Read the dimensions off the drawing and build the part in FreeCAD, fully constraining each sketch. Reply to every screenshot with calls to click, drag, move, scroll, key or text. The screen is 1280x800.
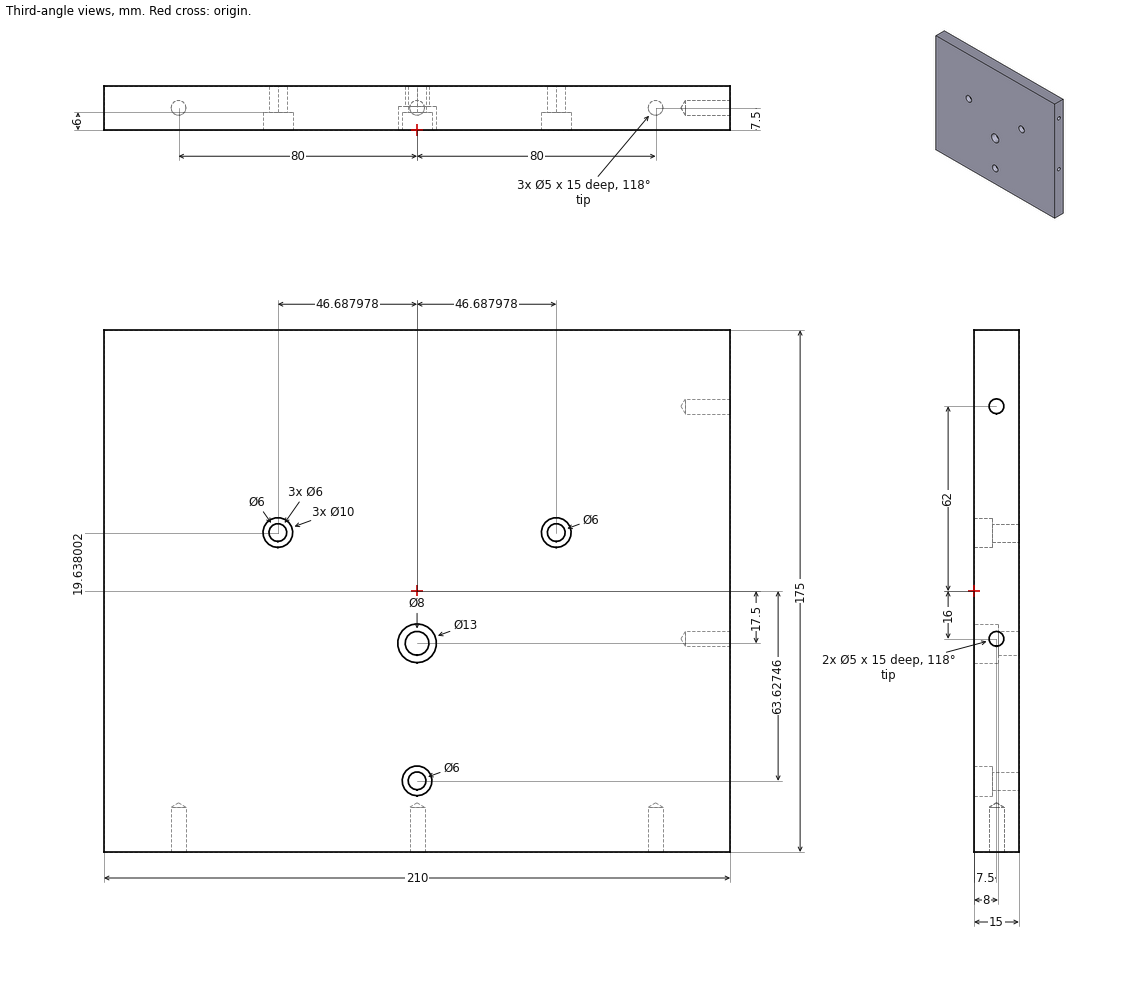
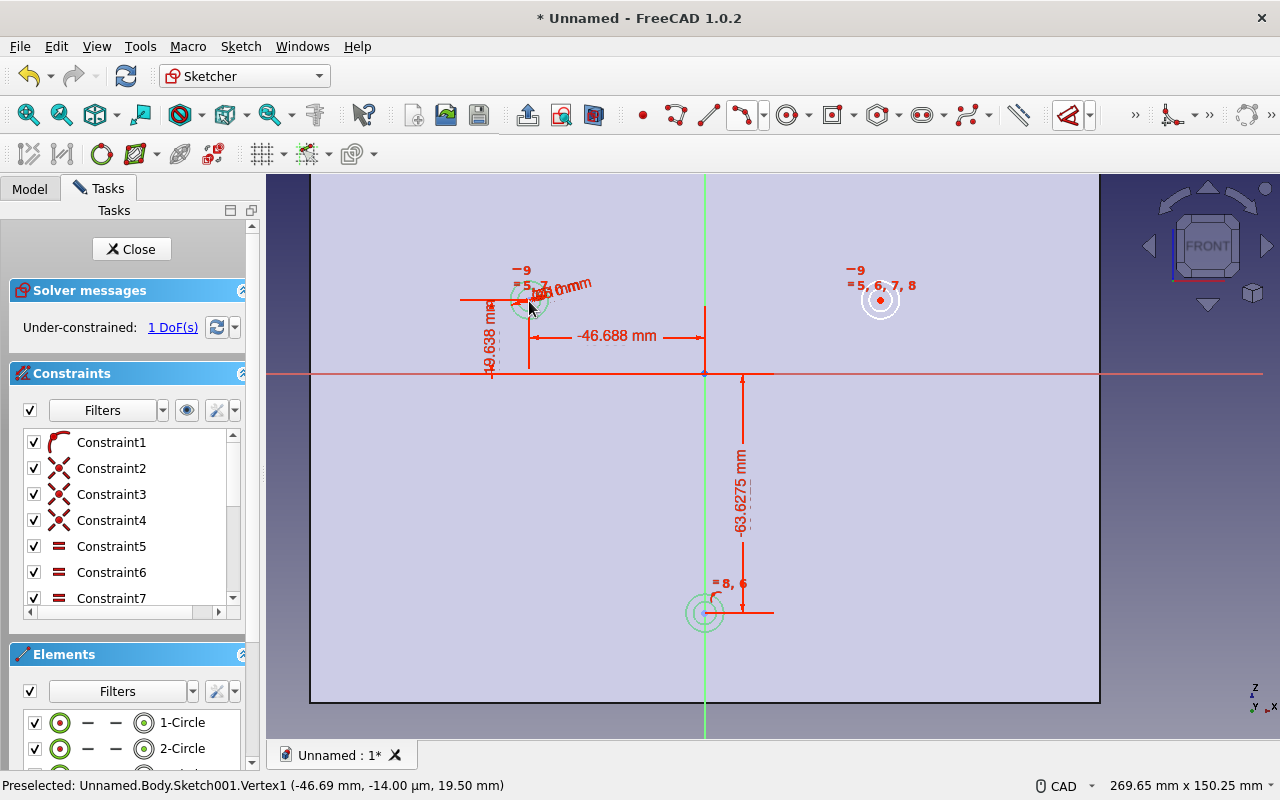
click(881, 300)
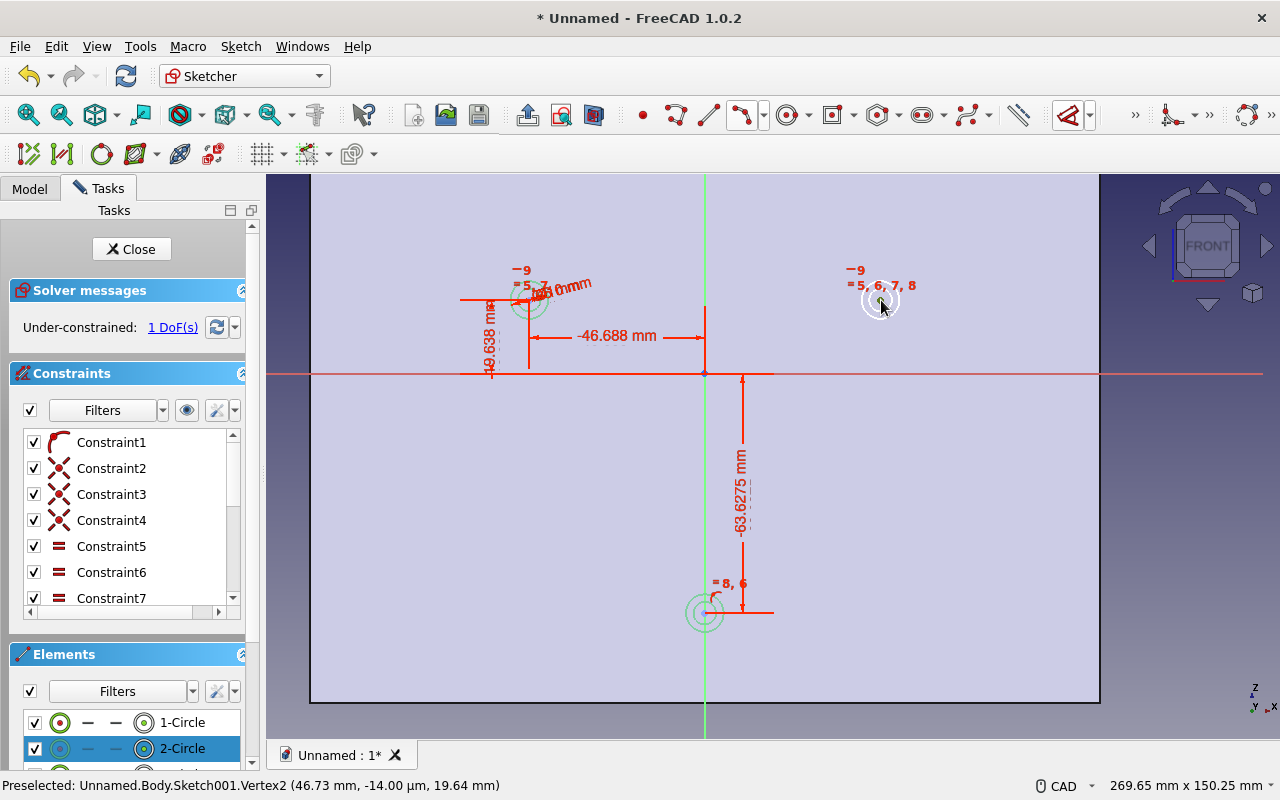
key(l)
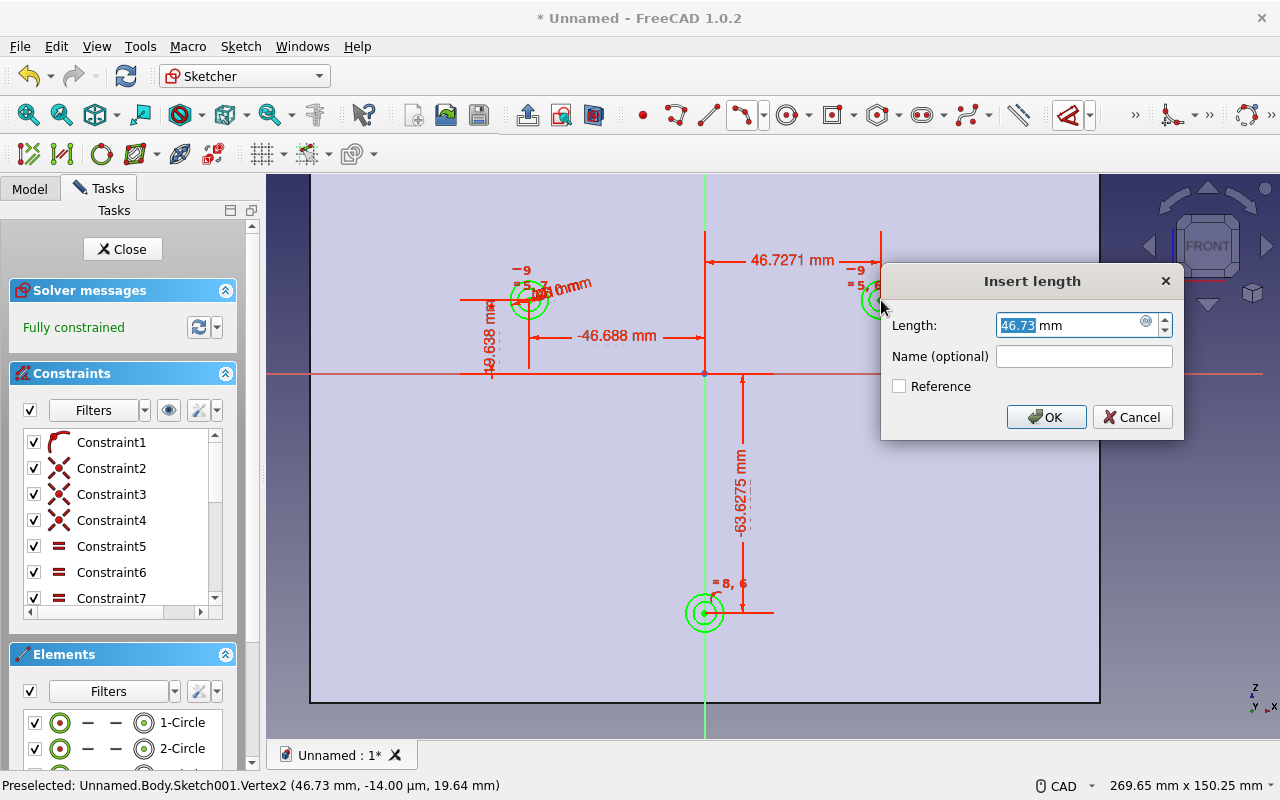
text(46.687978)
key(Return)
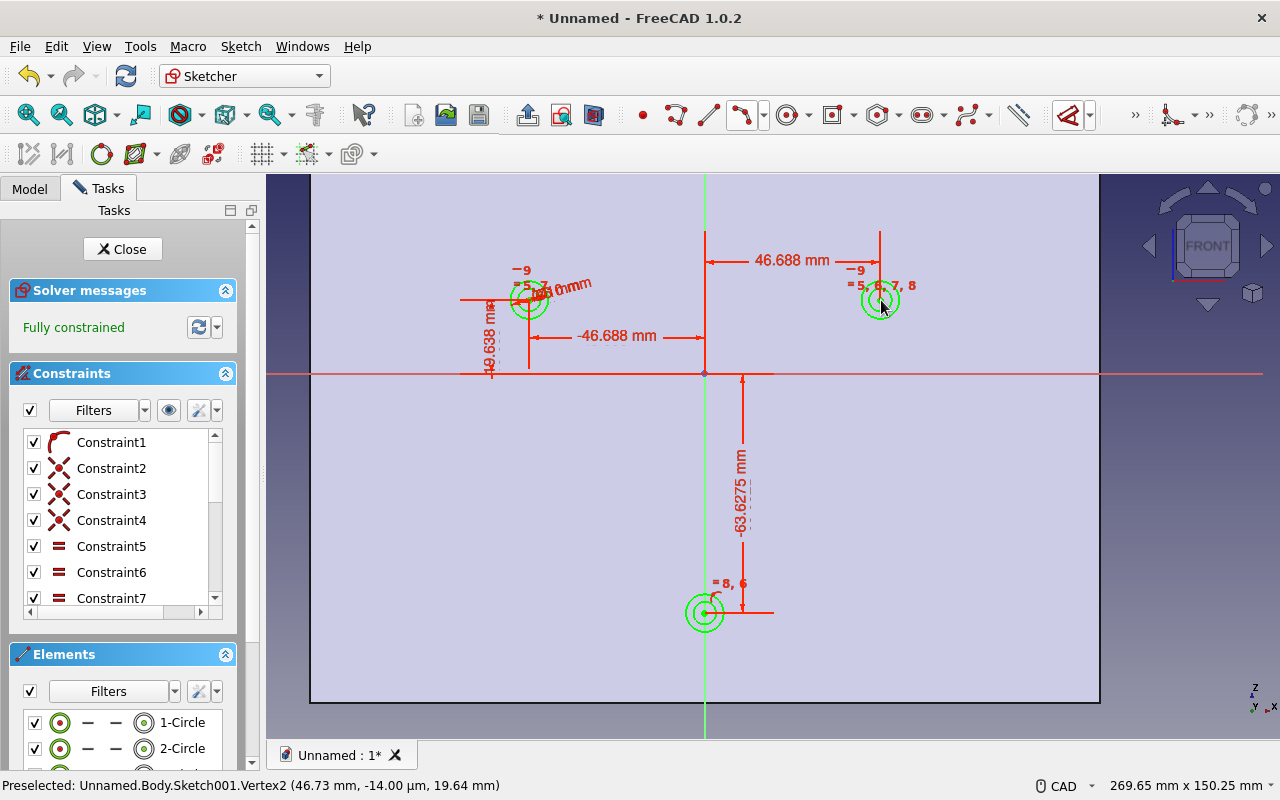
click(123, 249)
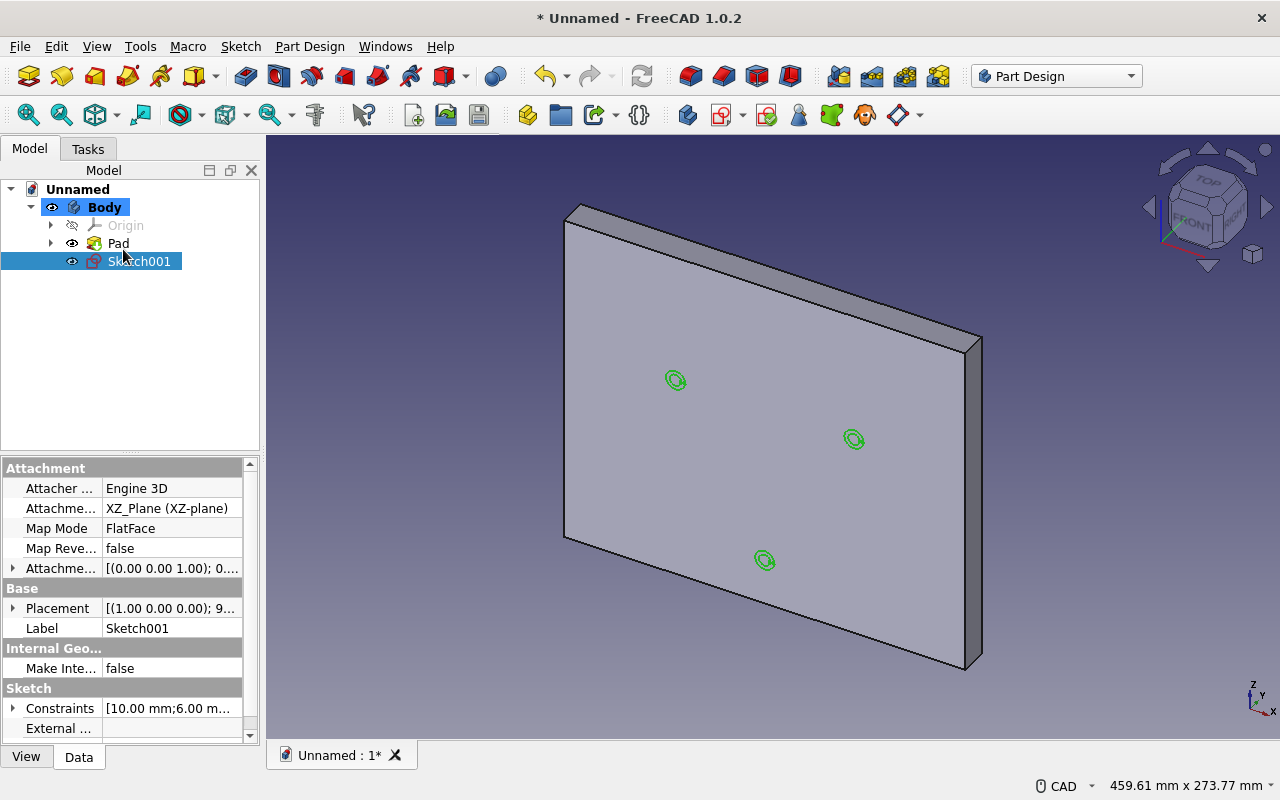
click(246, 76)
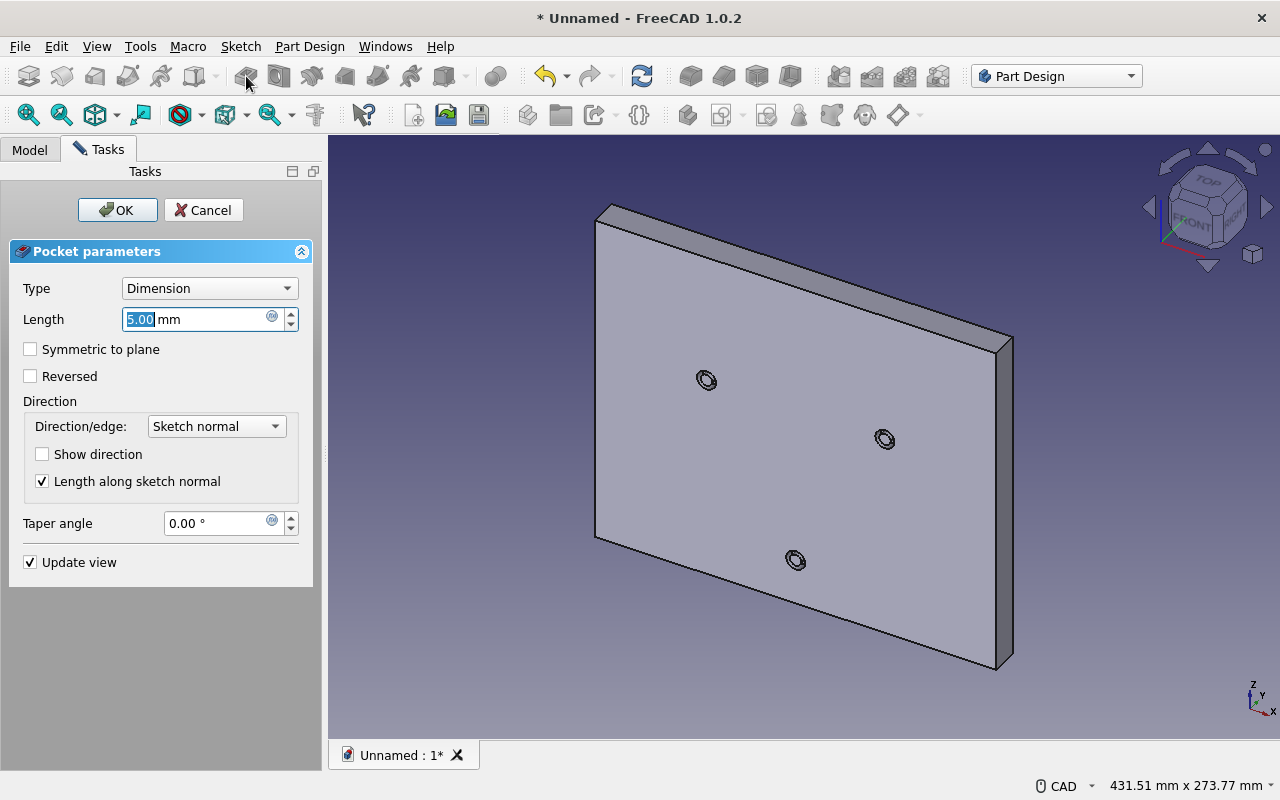
text(6)
key(Tab)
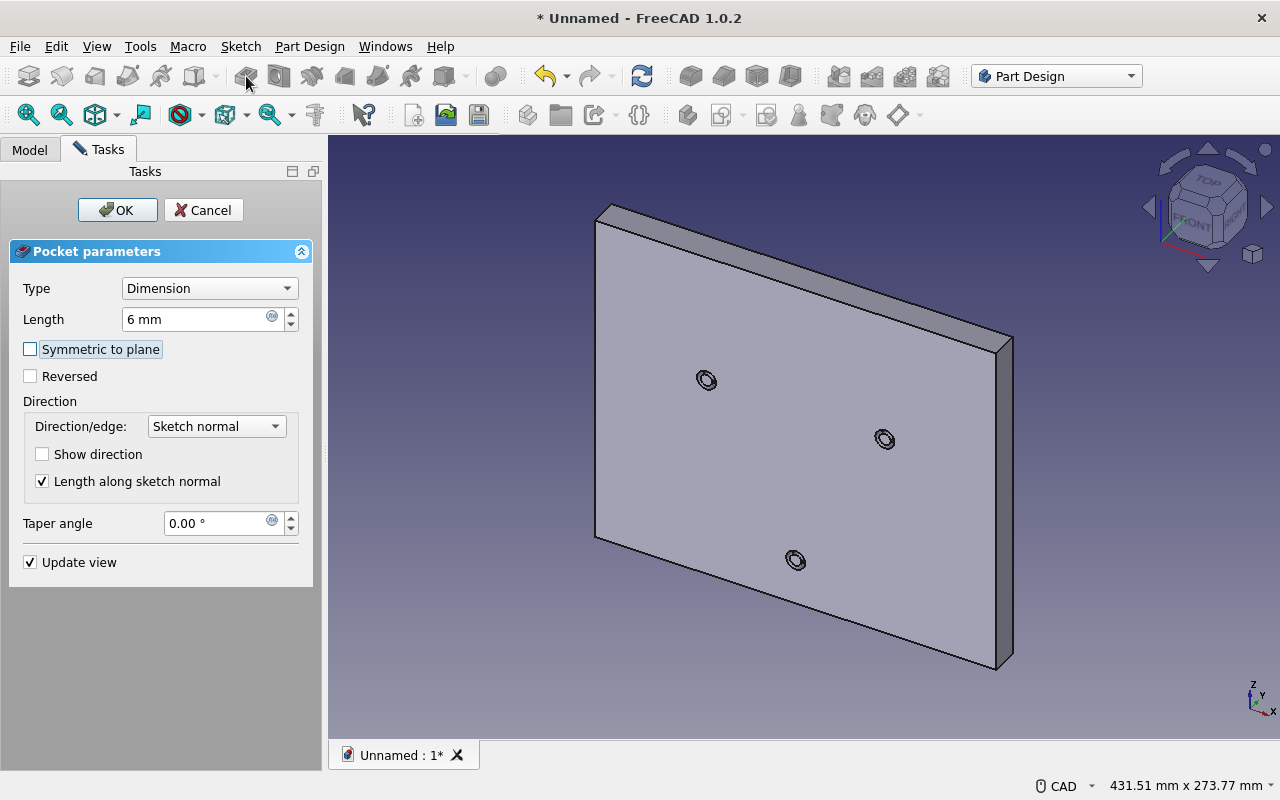
click(118, 210)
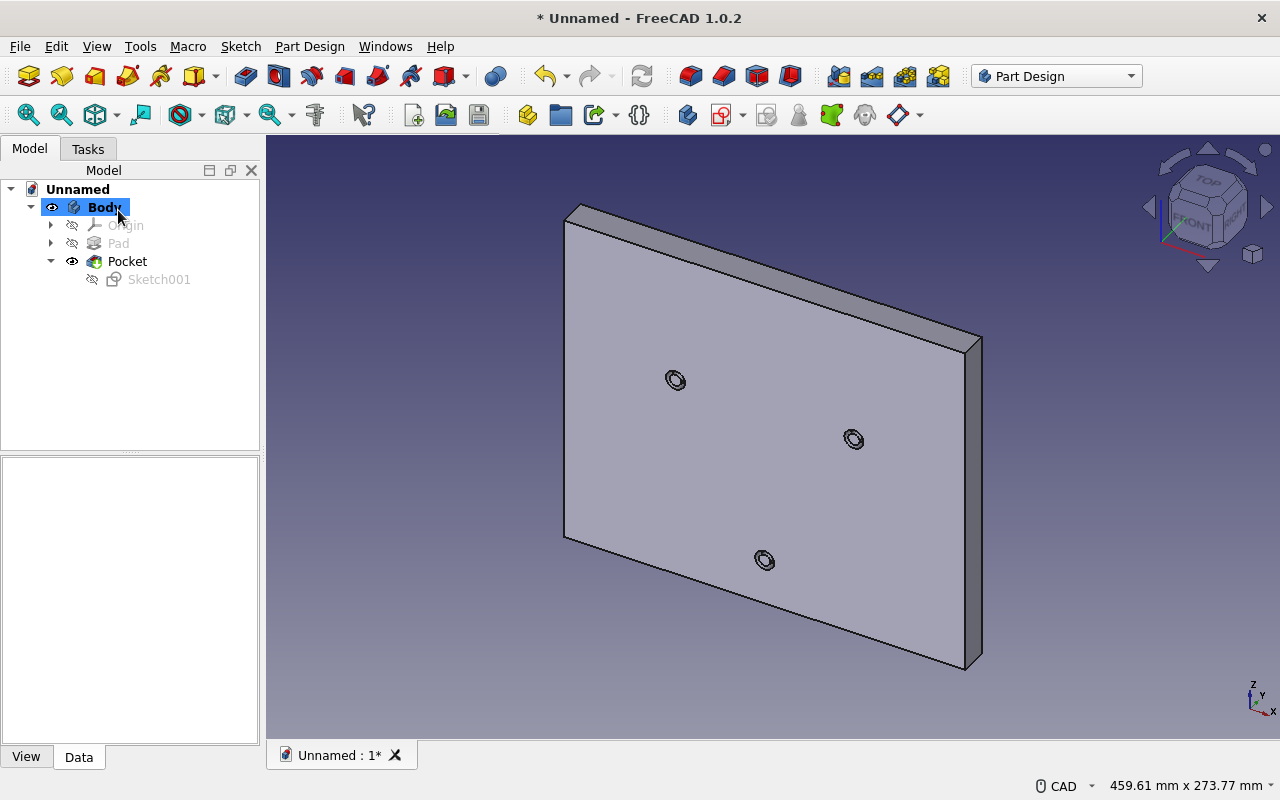
click(765, 444)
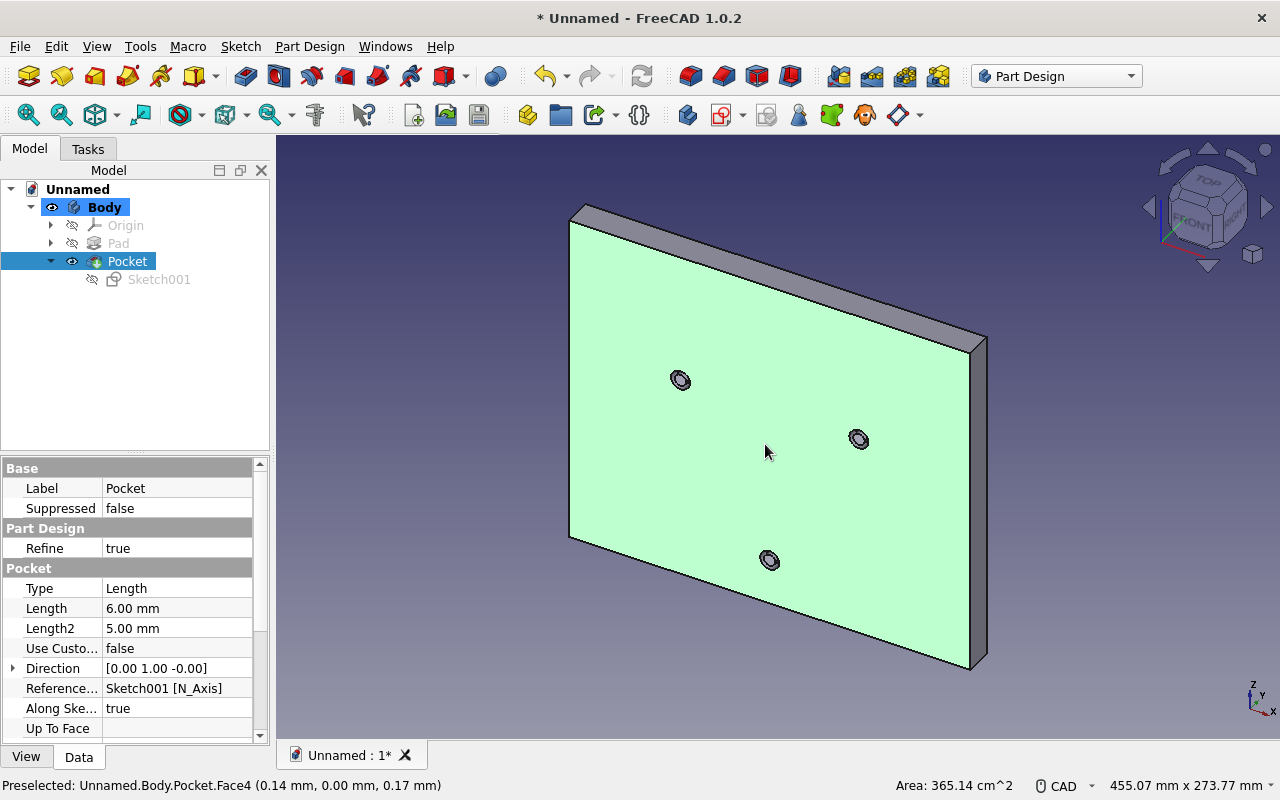
click(720, 116)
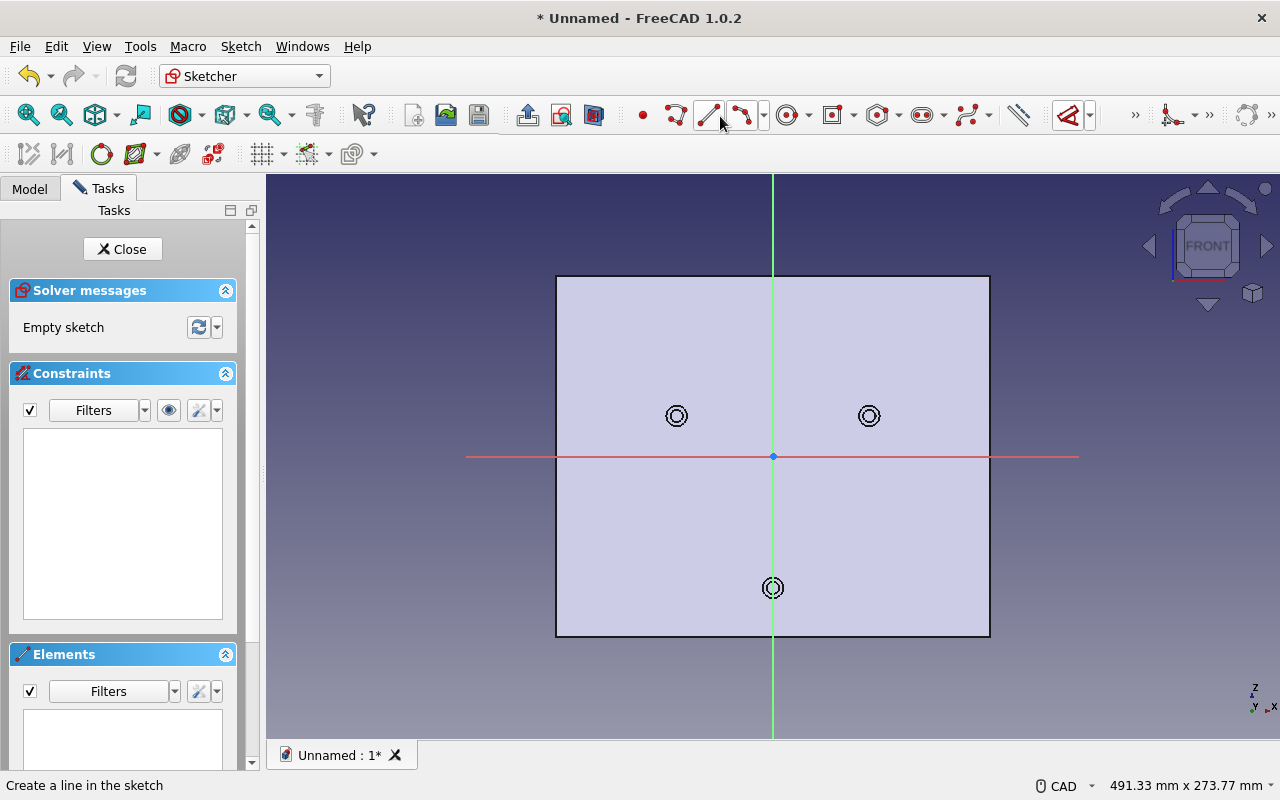
scroll(675, 414, up, 15)